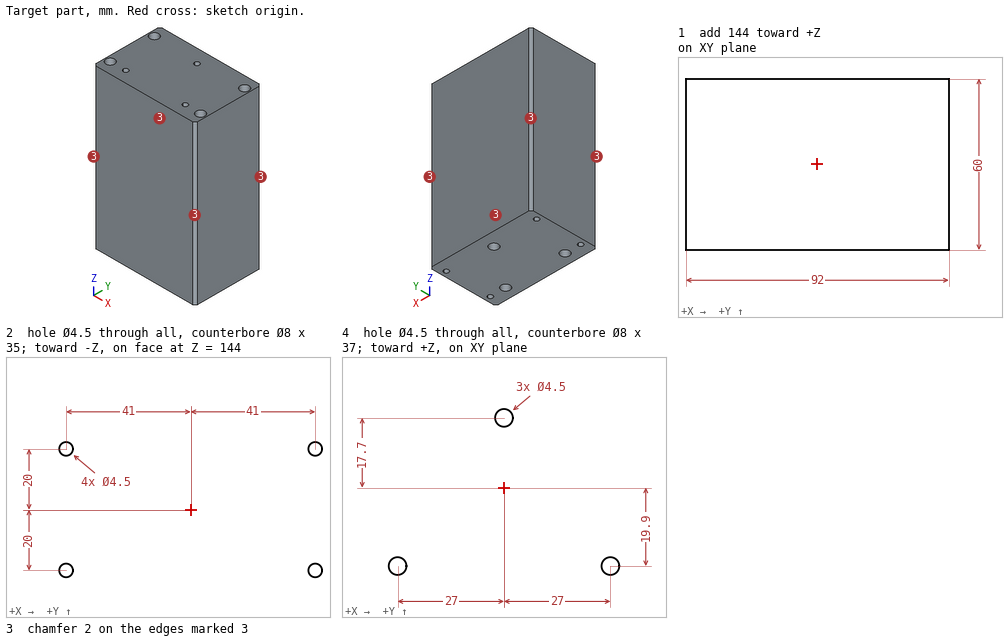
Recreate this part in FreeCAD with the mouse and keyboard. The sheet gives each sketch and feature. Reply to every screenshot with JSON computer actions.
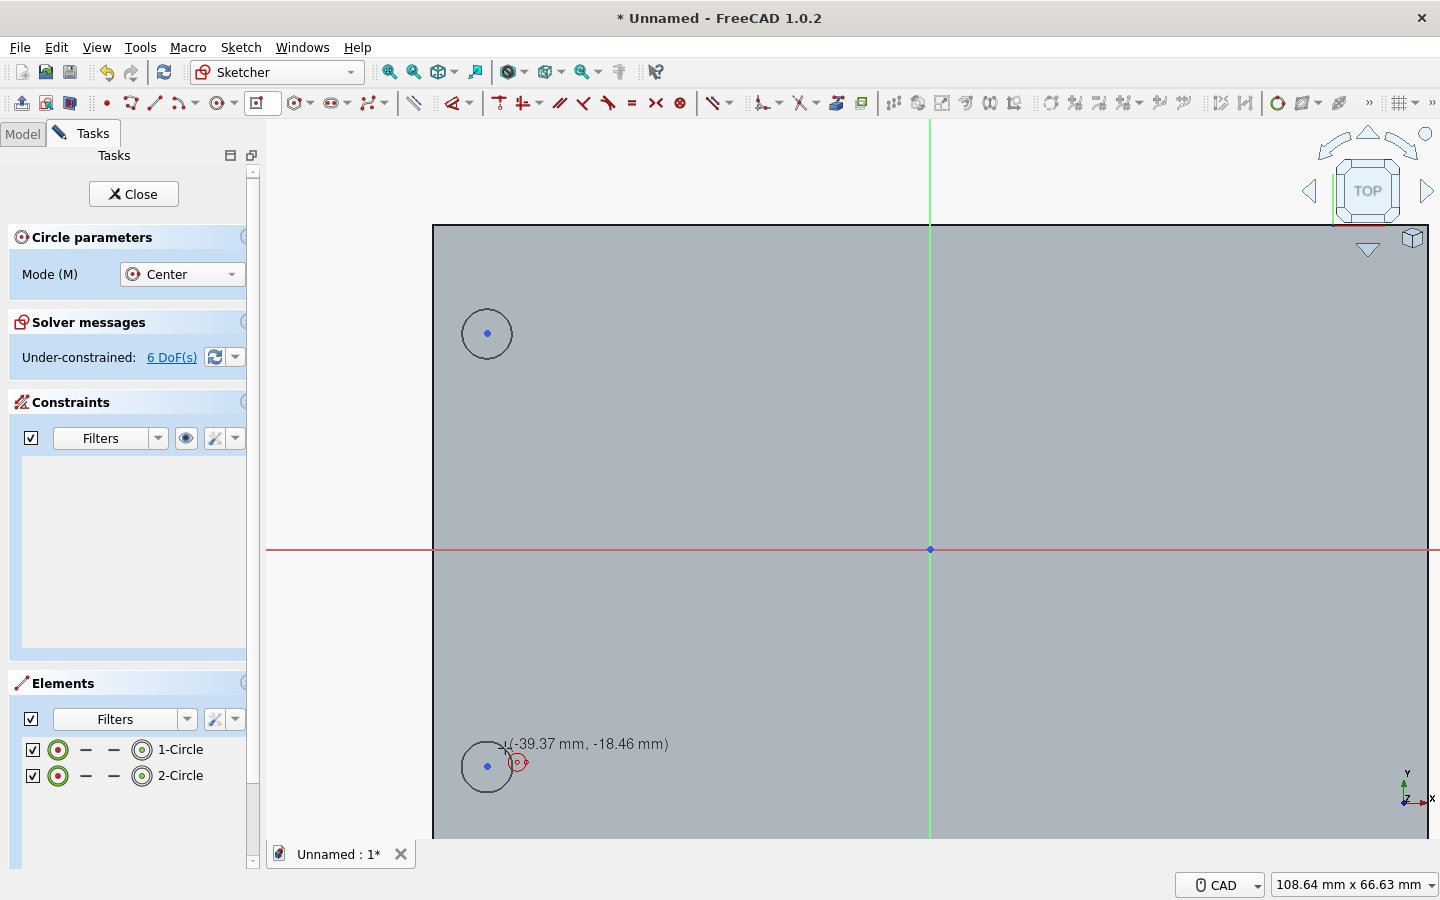
{"action": "scroll", "coordinate": [488, 336], "scroll_direction": "down", "scroll_amount": 2}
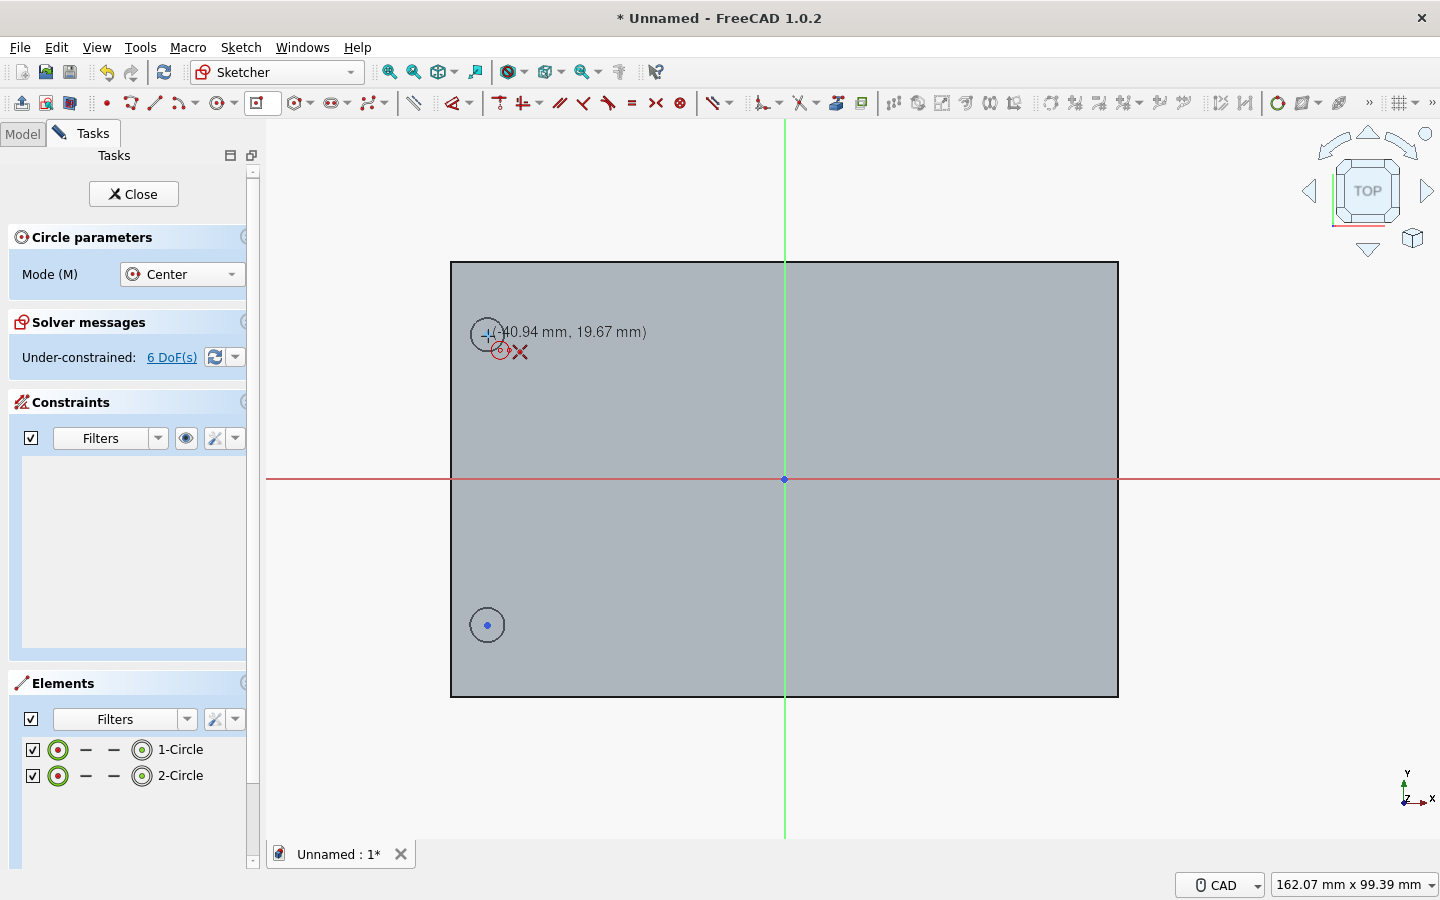
{"action": "scroll", "coordinate": [1082, 334], "scroll_direction": "up", "scroll_amount": 2}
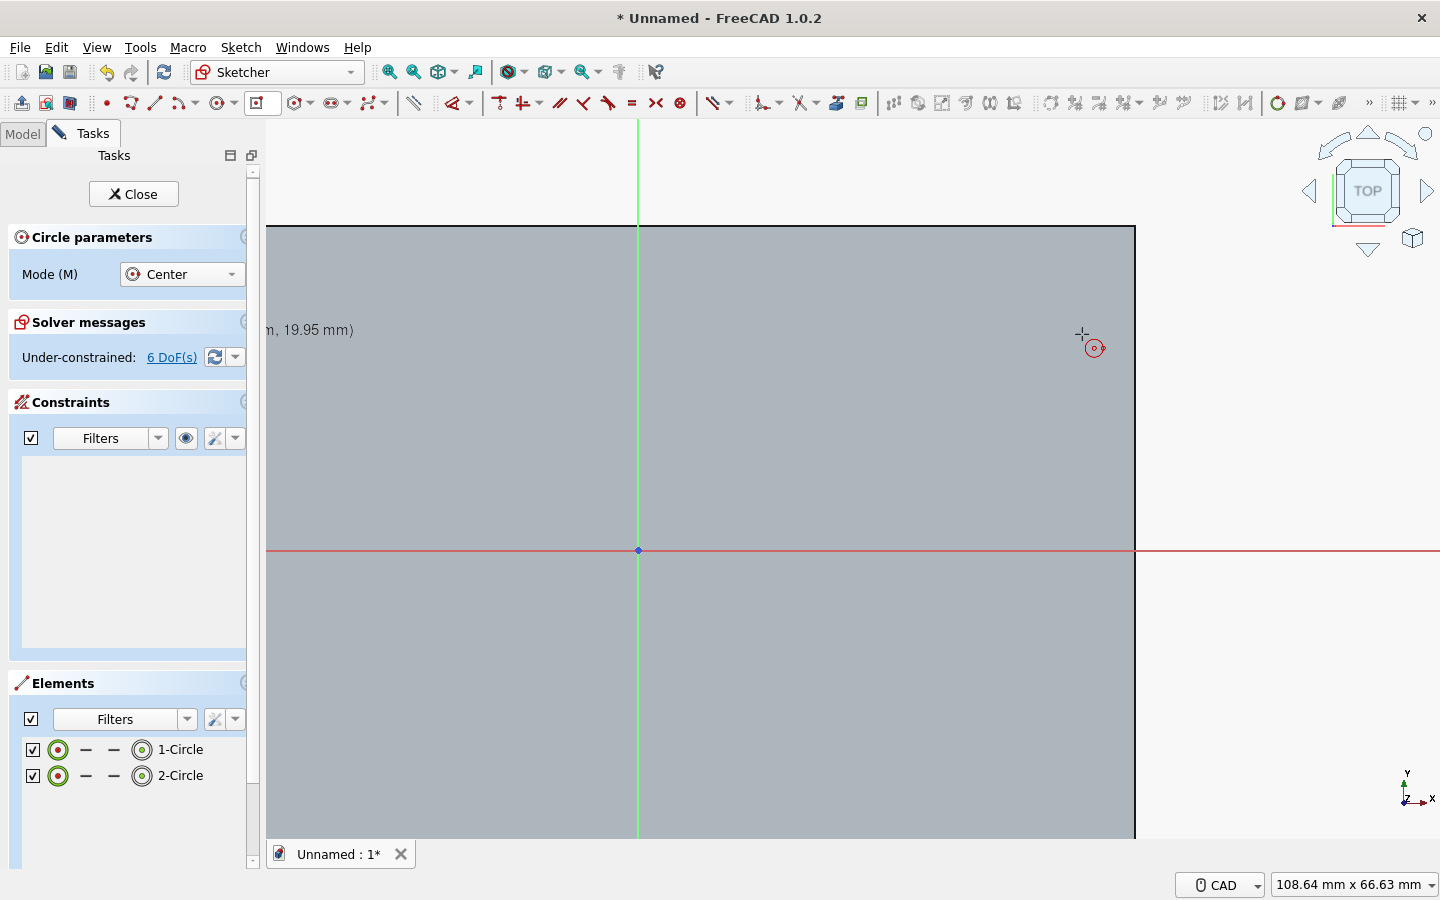
{"action": "left_click", "coordinate": [1081, 334]}
{"action": "left_click", "coordinate": [1098, 317]}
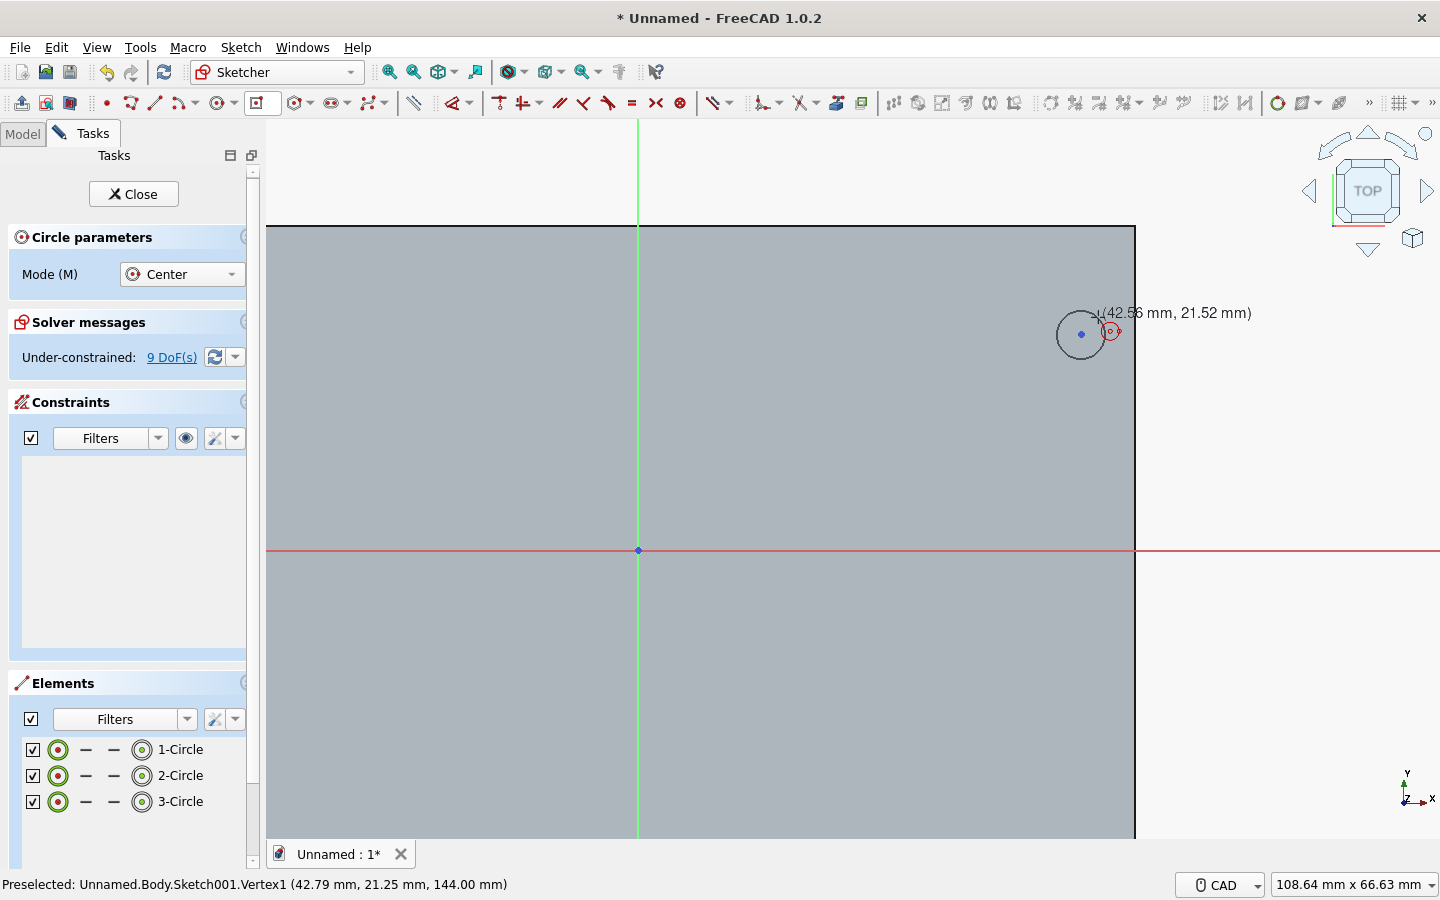
{"action": "left_click", "coordinate": [1081, 767]}
{"action": "left_click", "coordinate": [1098, 749]}
{"action": "key", "text": "Escape"}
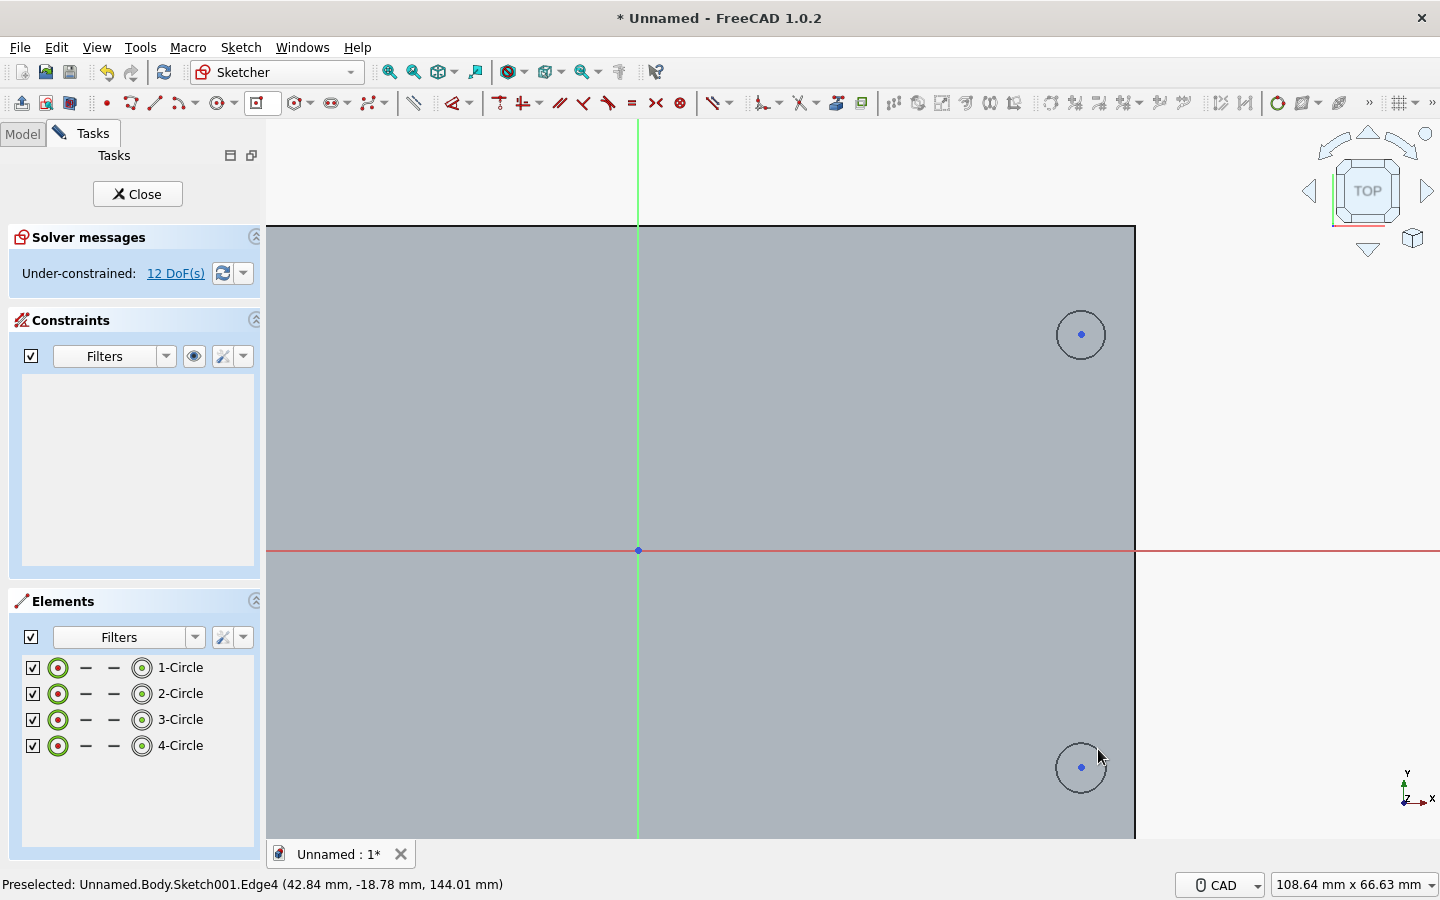
{"action": "scroll", "coordinate": [1082, 334], "scroll_direction": "down", "scroll_amount": 2}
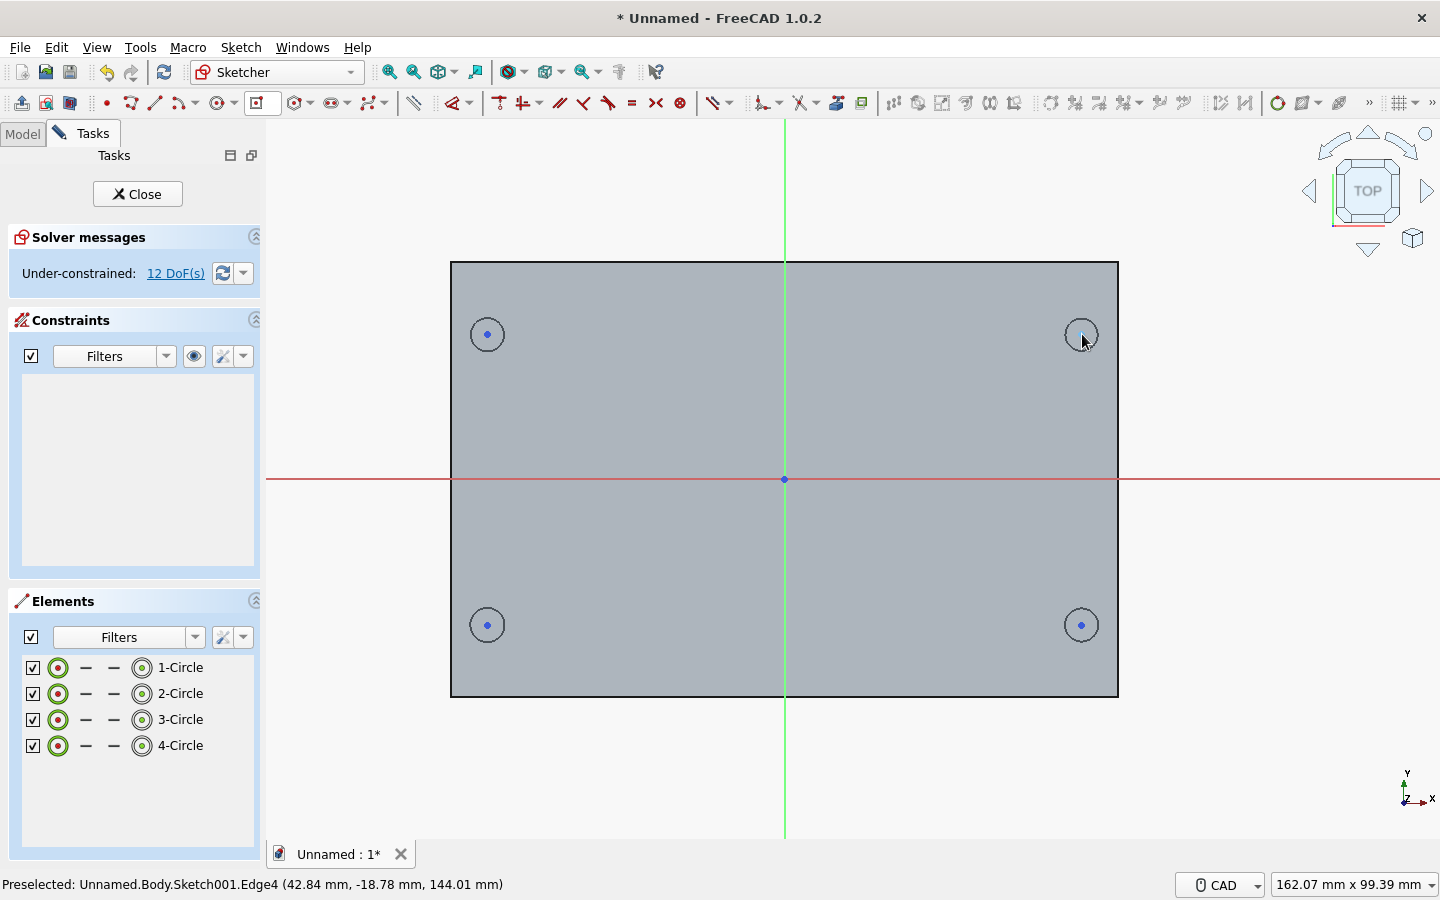
{"action": "left_click", "coordinate": [499, 323]}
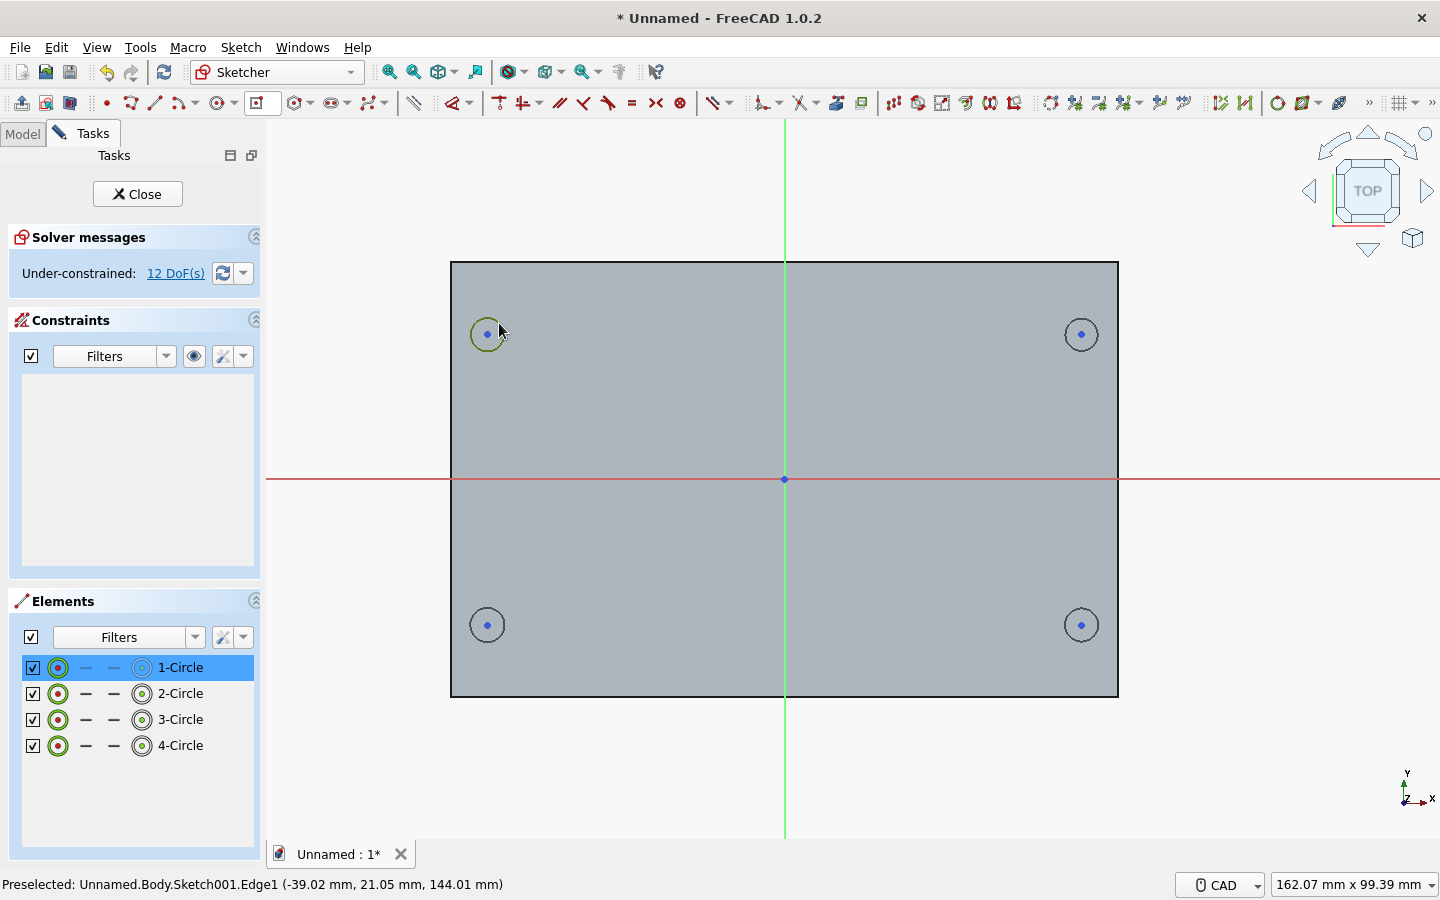
{"action": "left_click", "coordinate": [499, 613]}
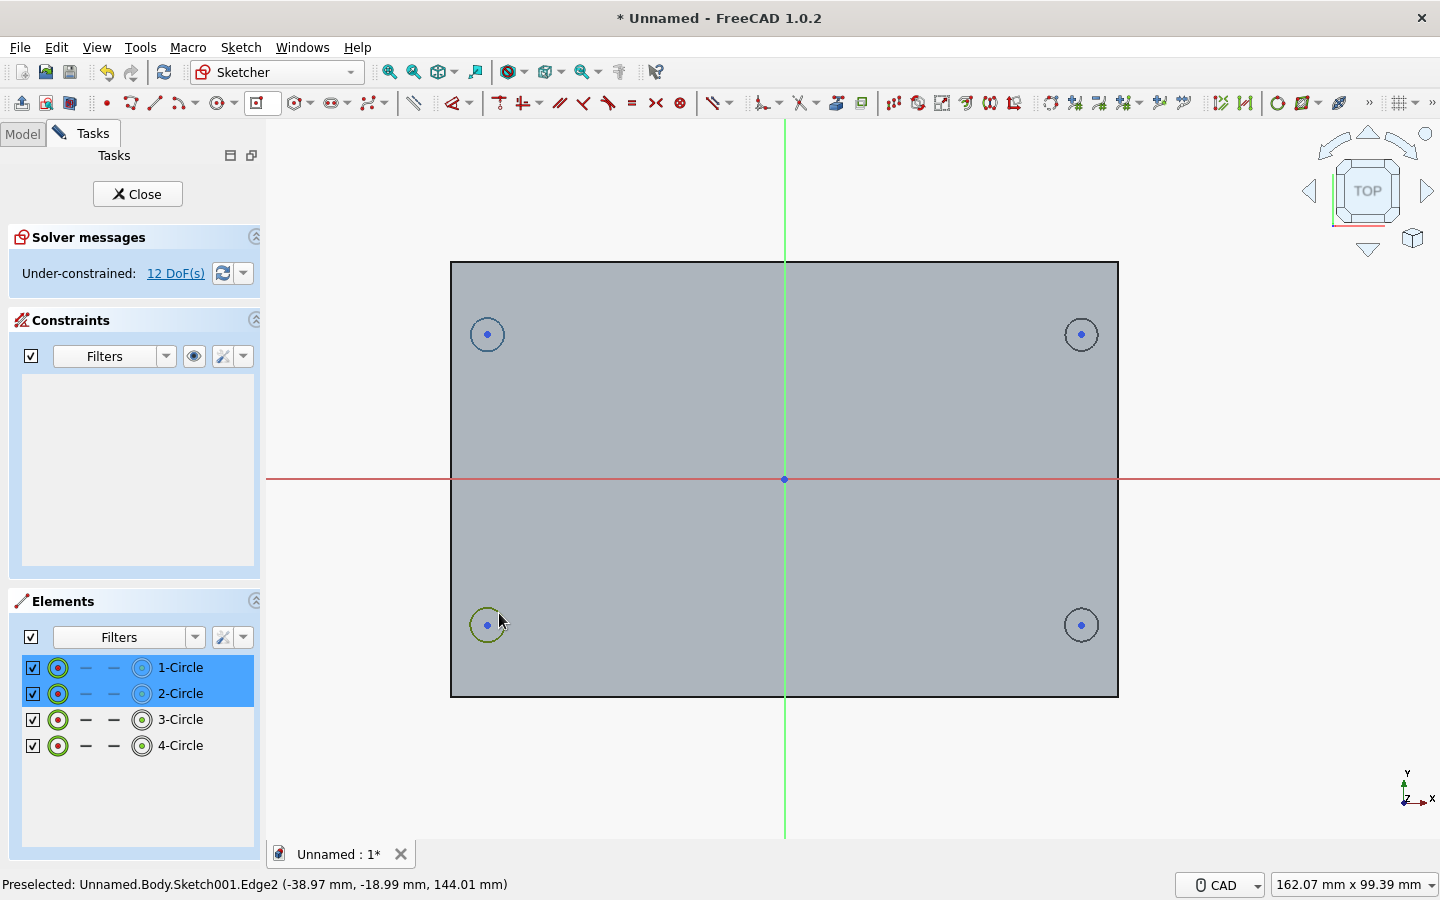
{"action": "left_click", "coordinate": [1093, 323]}